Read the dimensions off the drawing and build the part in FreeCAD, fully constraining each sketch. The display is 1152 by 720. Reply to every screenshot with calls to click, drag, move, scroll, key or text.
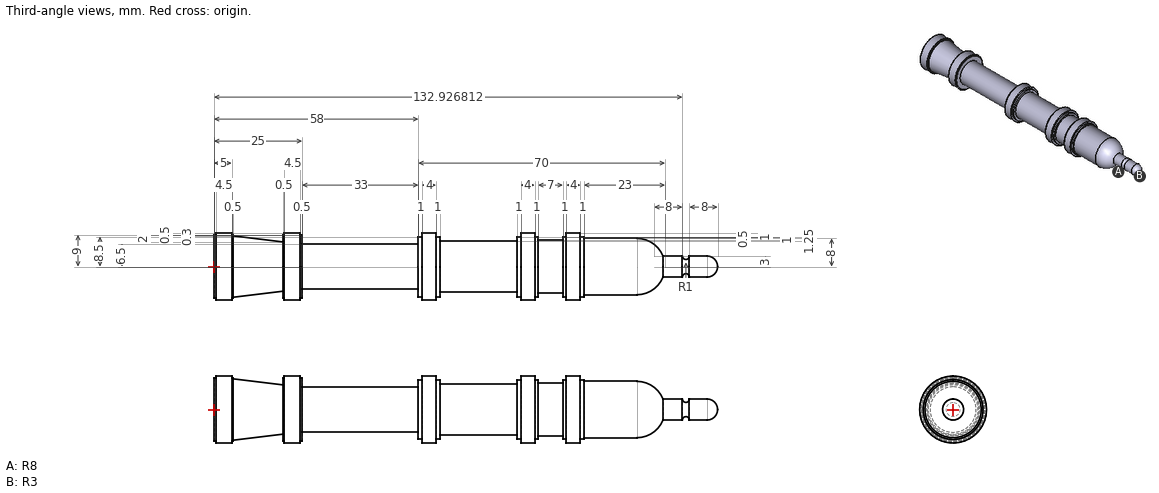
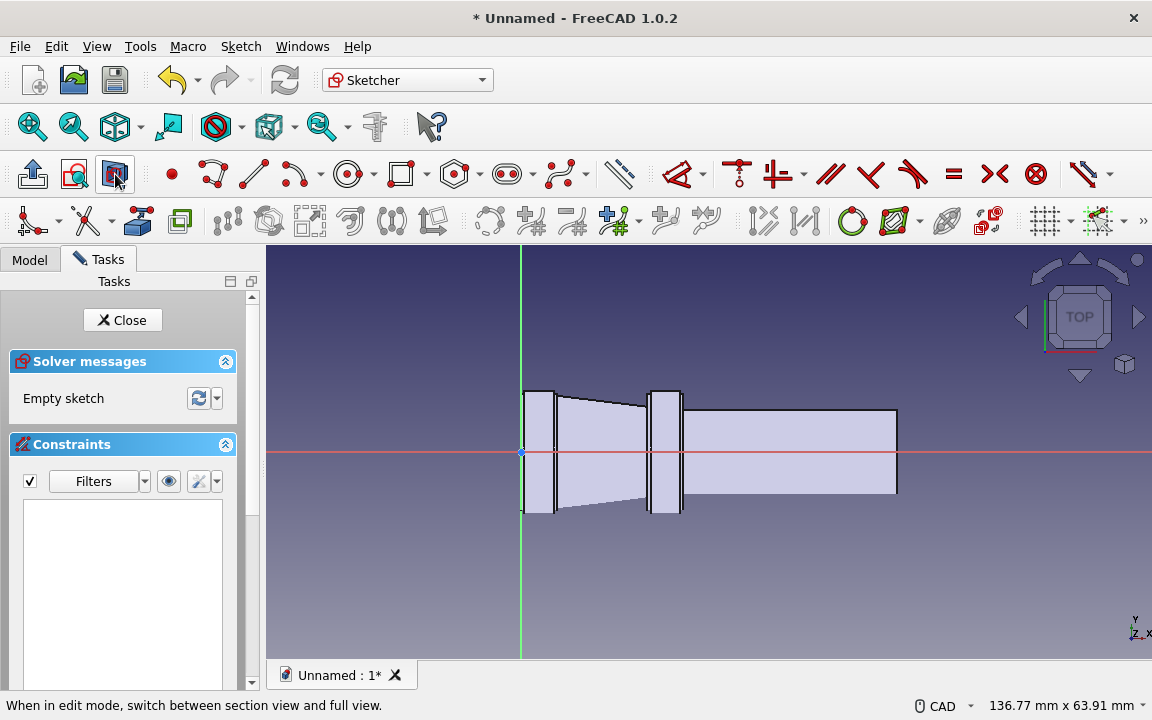
scroll(294, 489, down, 3)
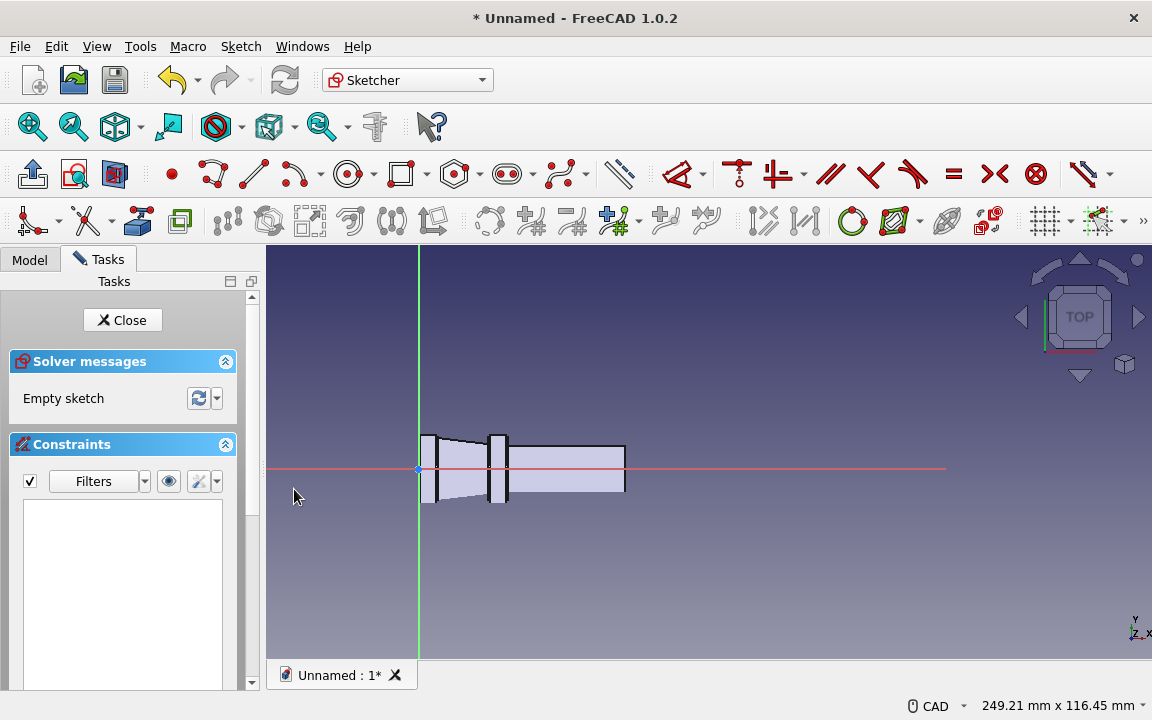
click(213, 174)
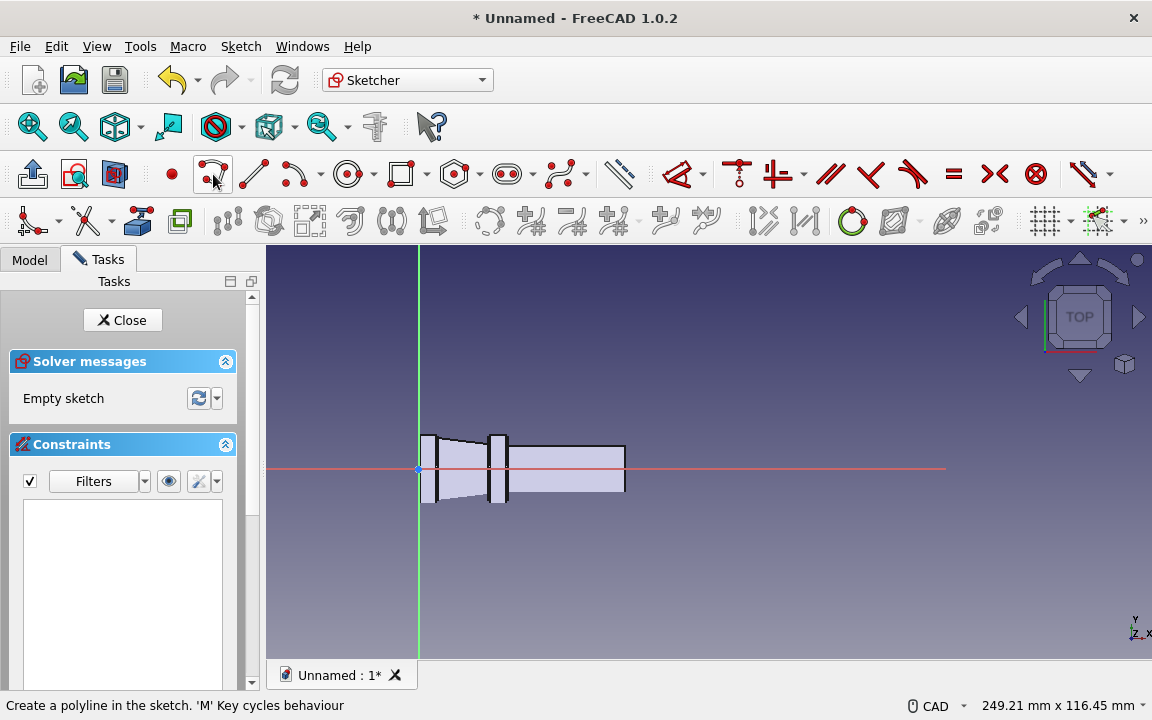
click(625, 469)
click(874, 460)
click(874, 441)
click(792, 441)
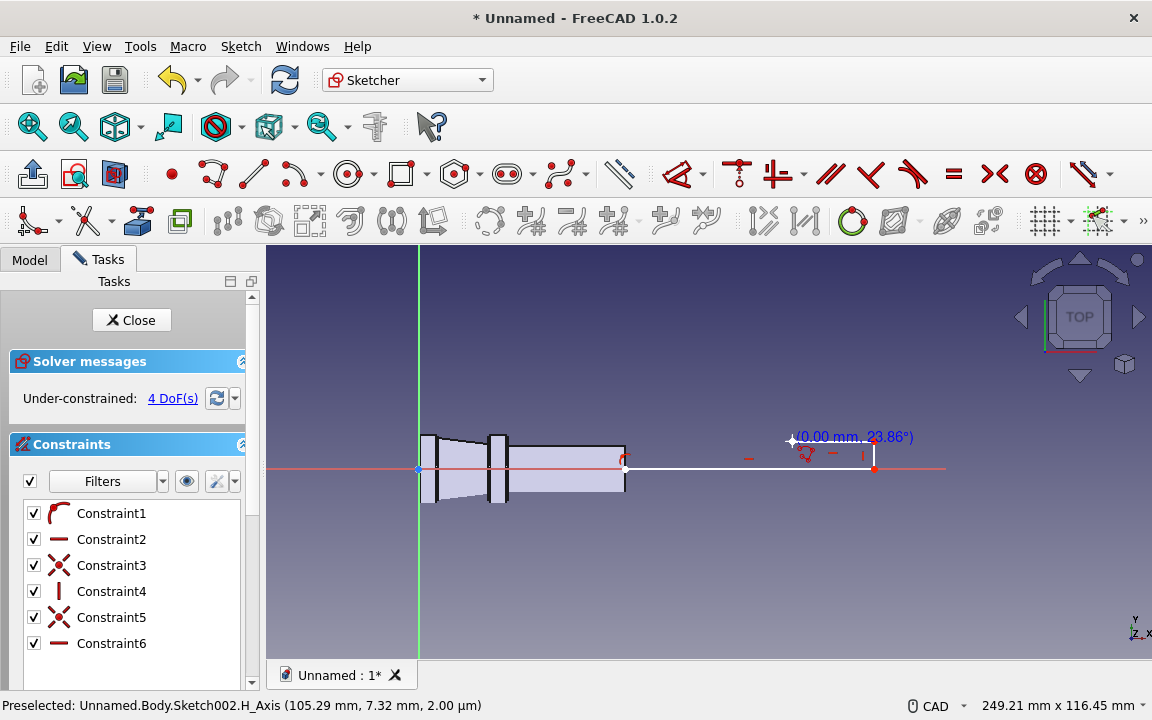
scroll(792, 439, up, 11)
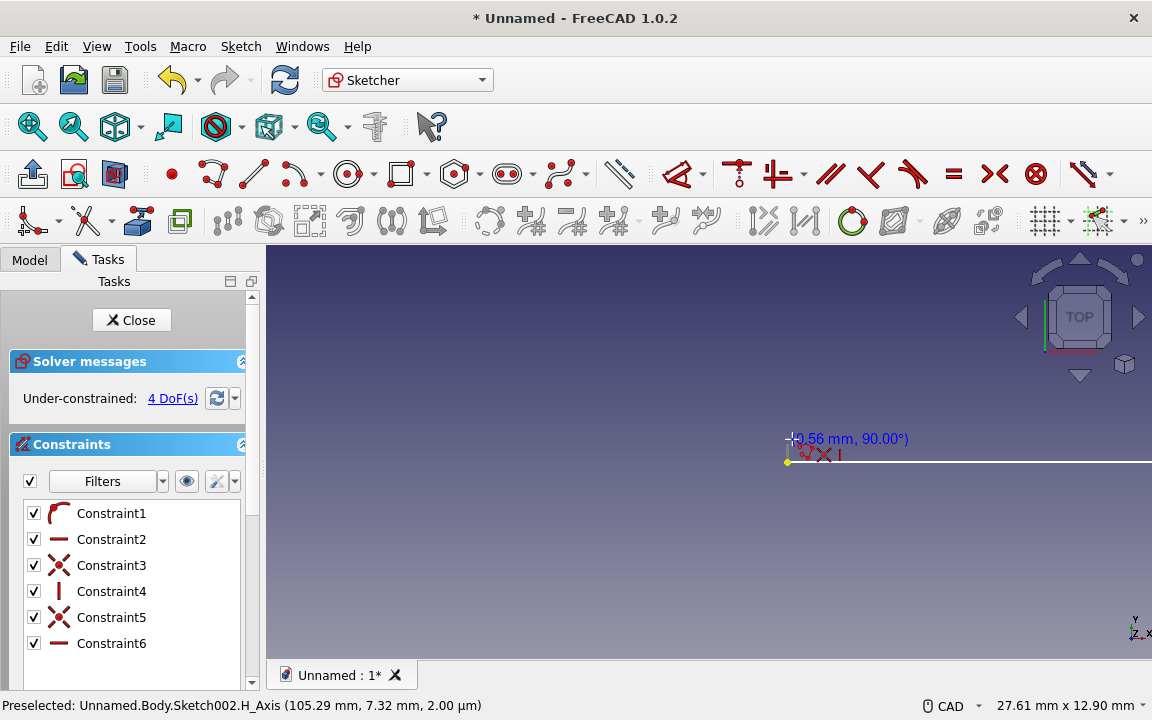
click(787, 433)
click(755, 433)
click(755, 401)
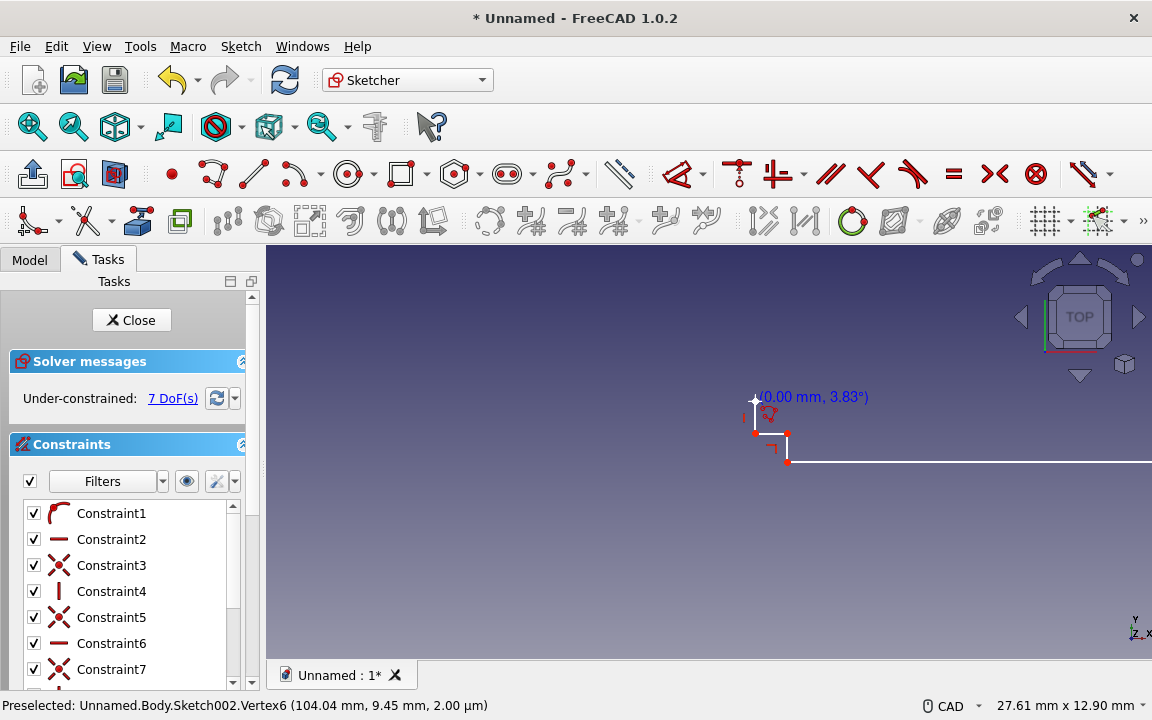
scroll(786, 439, down, 11)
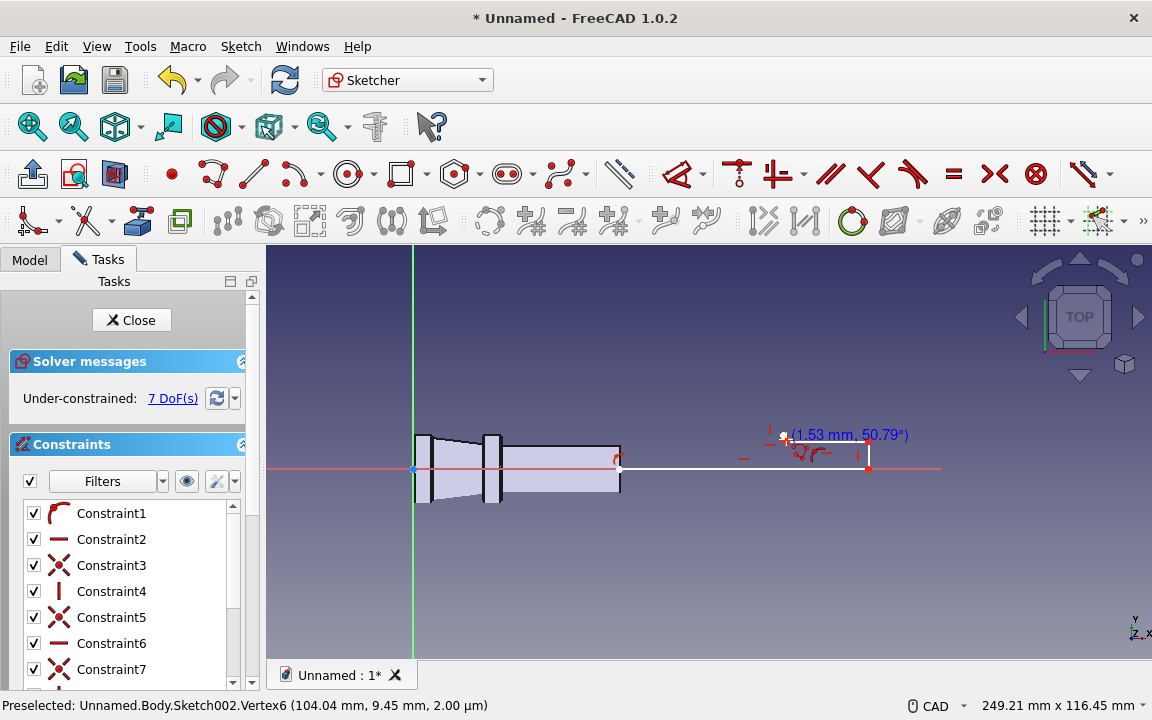
click(769, 435)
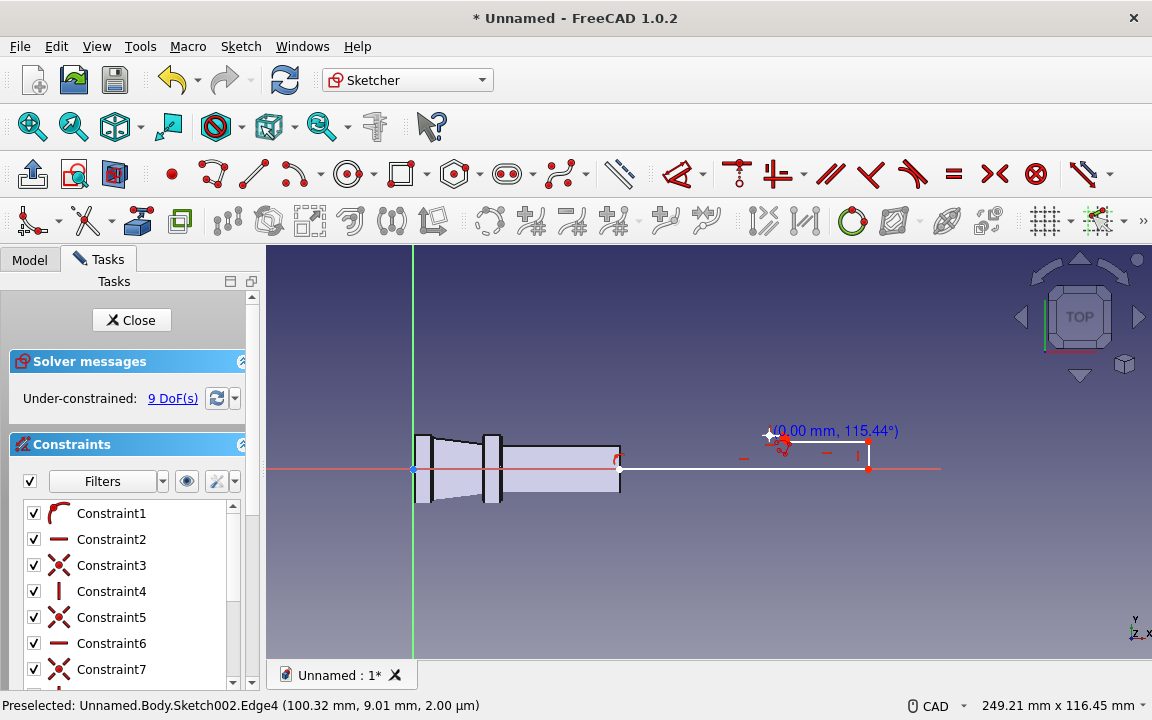
scroll(769, 439, up, 8)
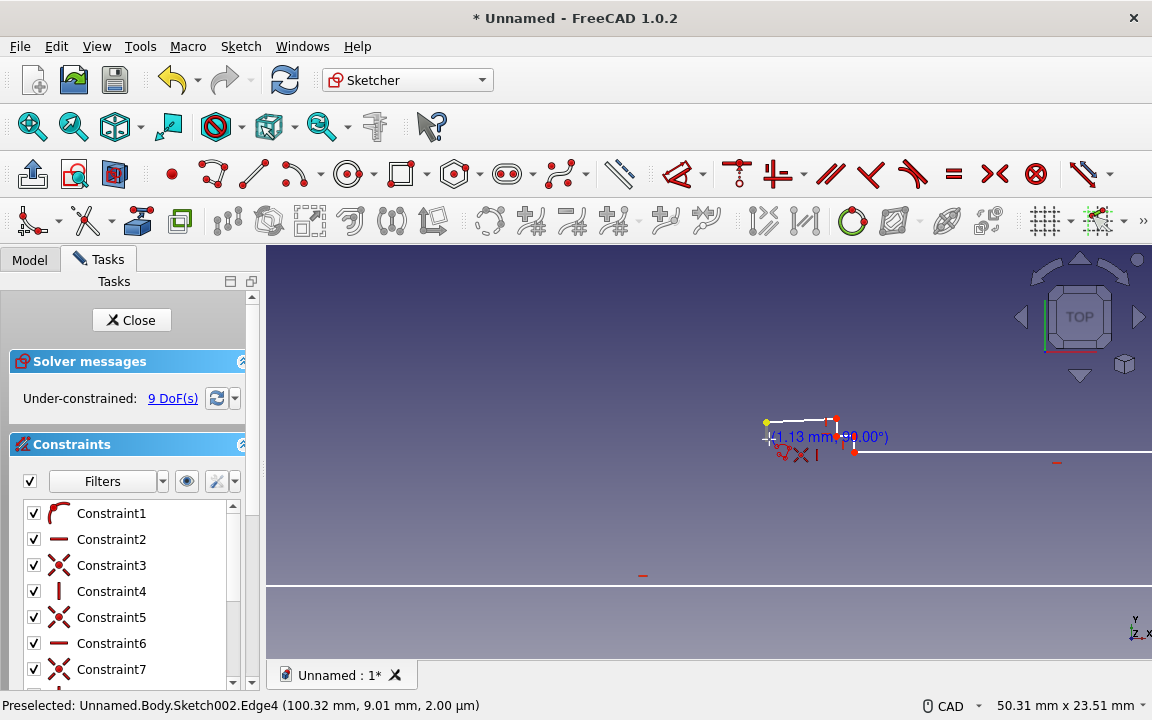
click(767, 436)
click(748, 436)
click(748, 454)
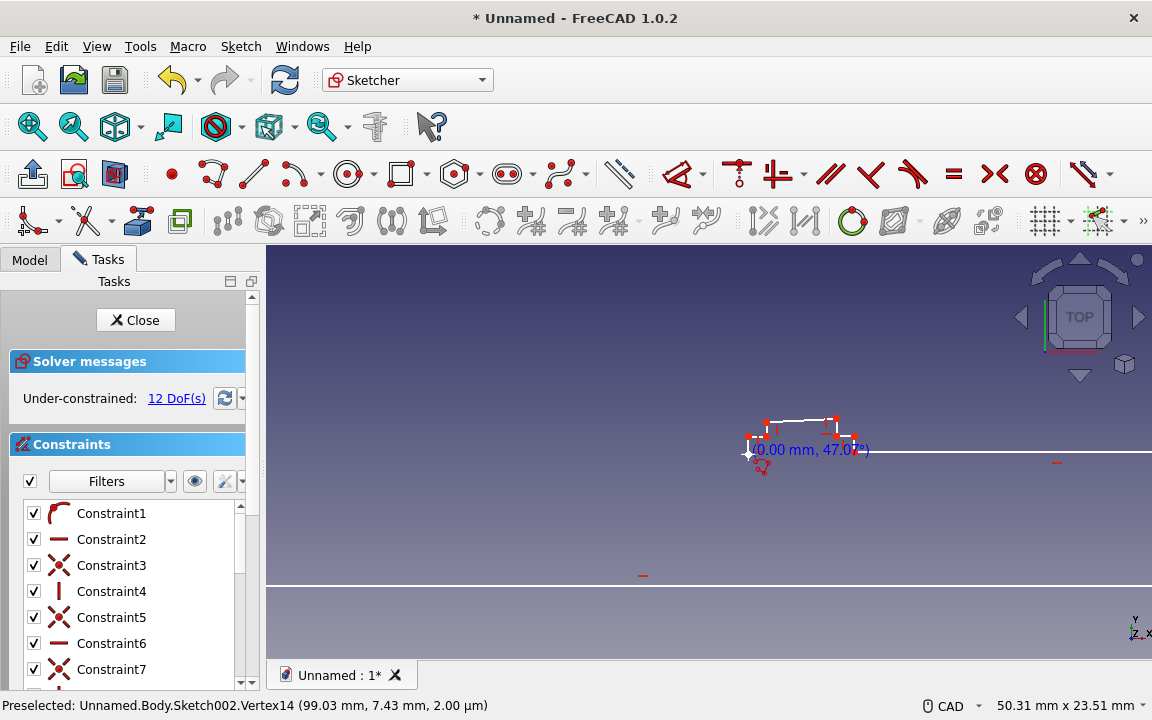
scroll(769, 439, down, 8)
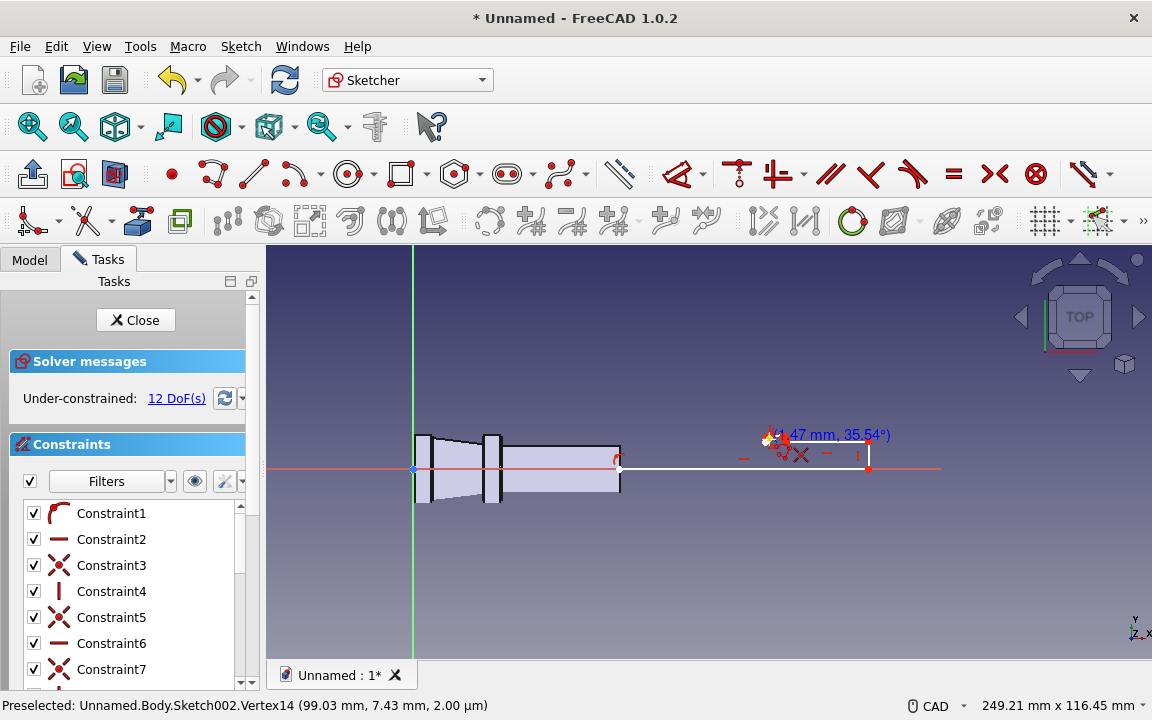
click(740, 442)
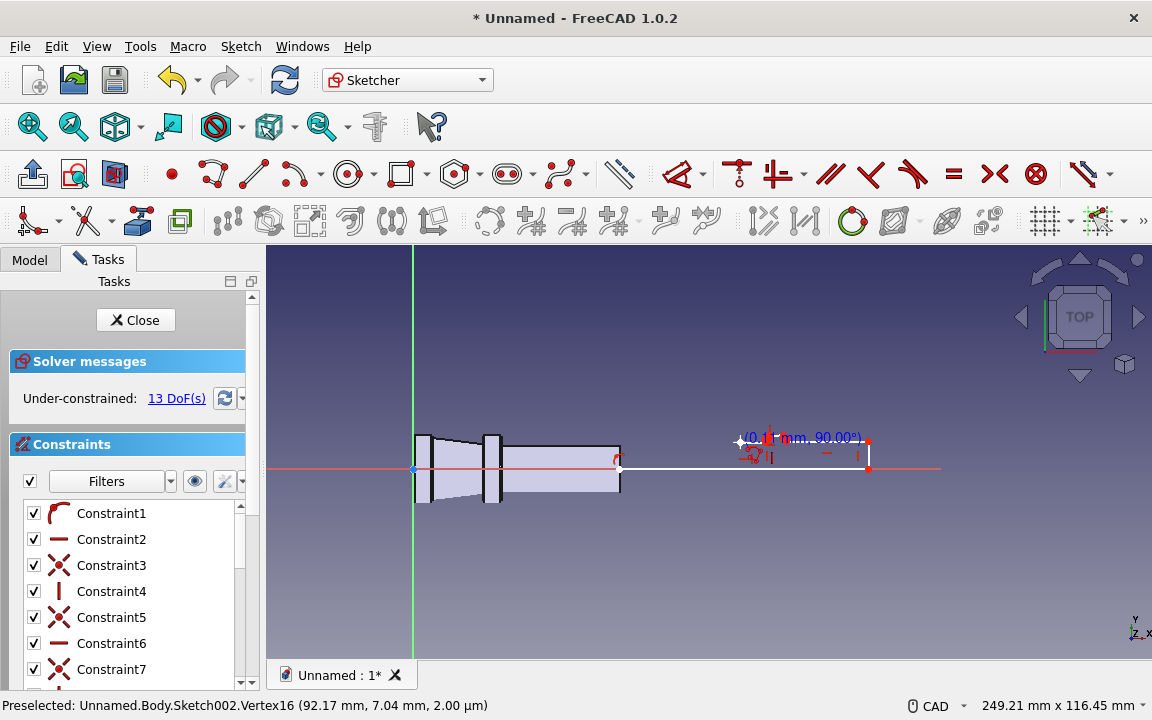
scroll(740, 439, up, 8)